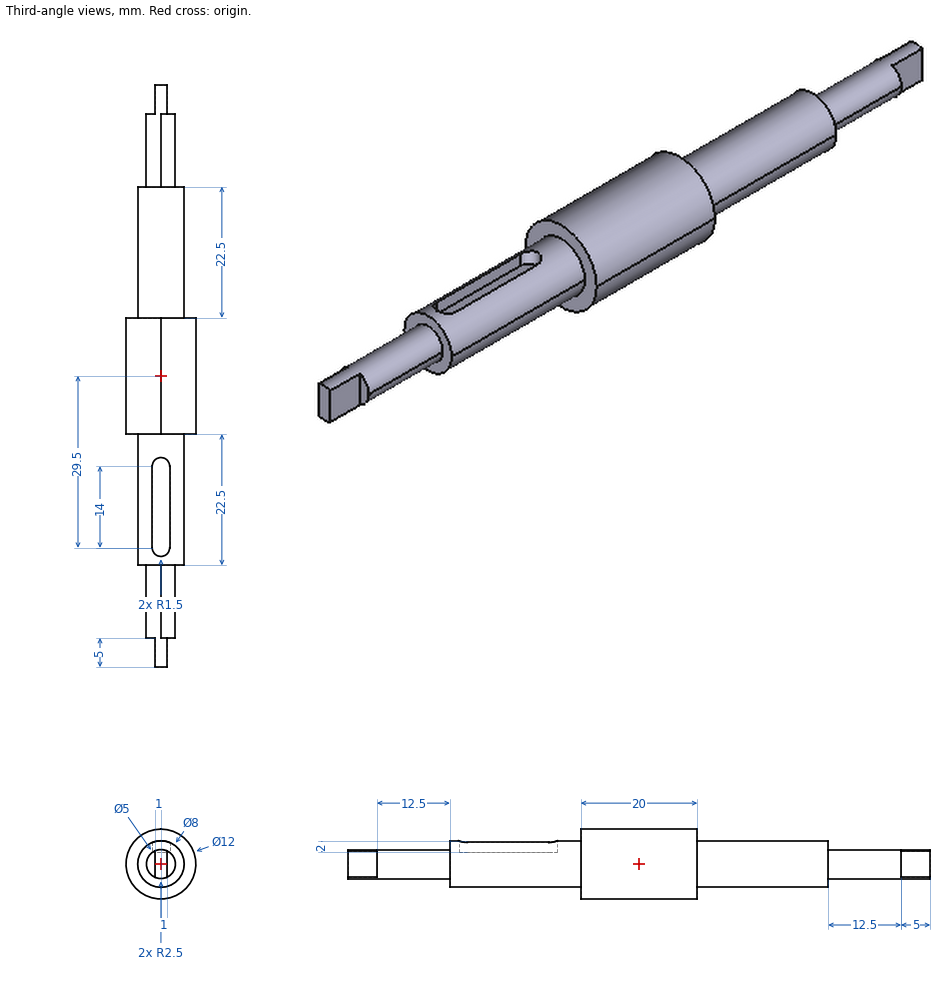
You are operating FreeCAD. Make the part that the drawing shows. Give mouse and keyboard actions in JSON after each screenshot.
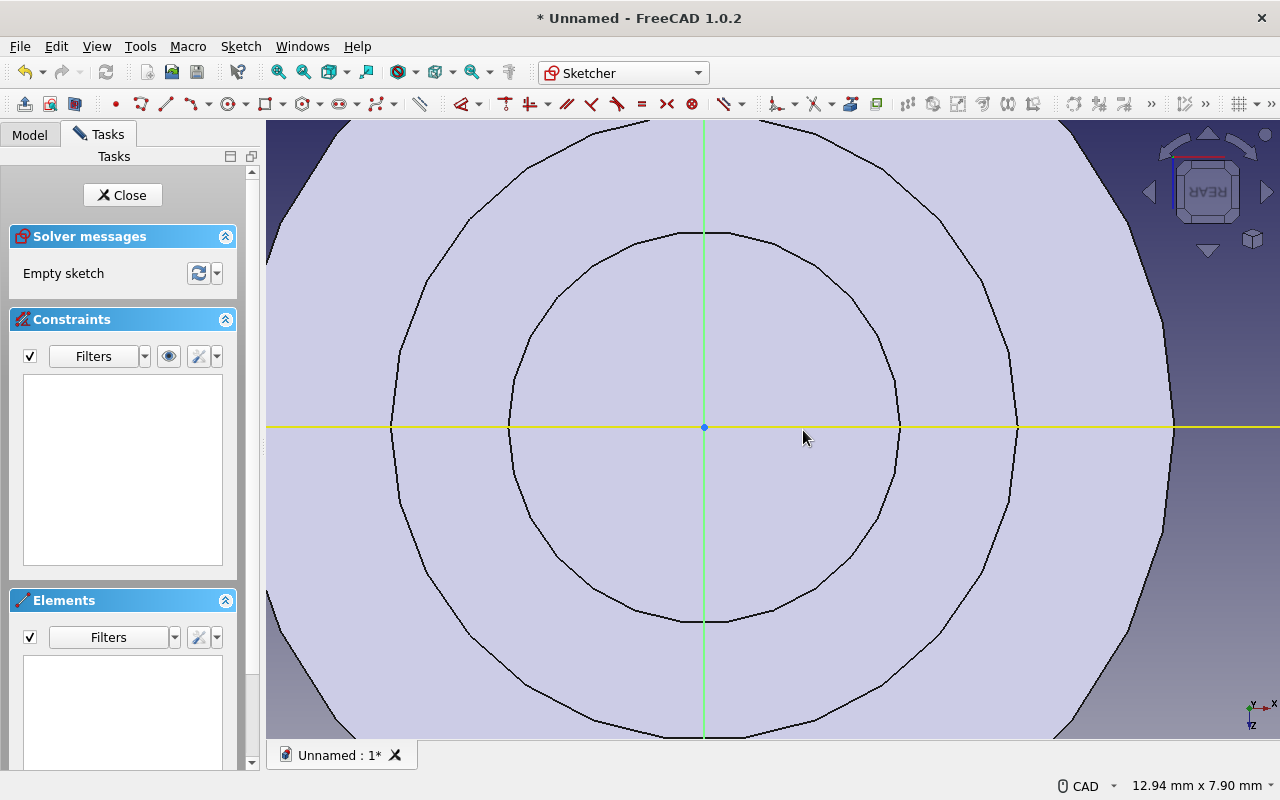
{"action": "key", "text": "g l"}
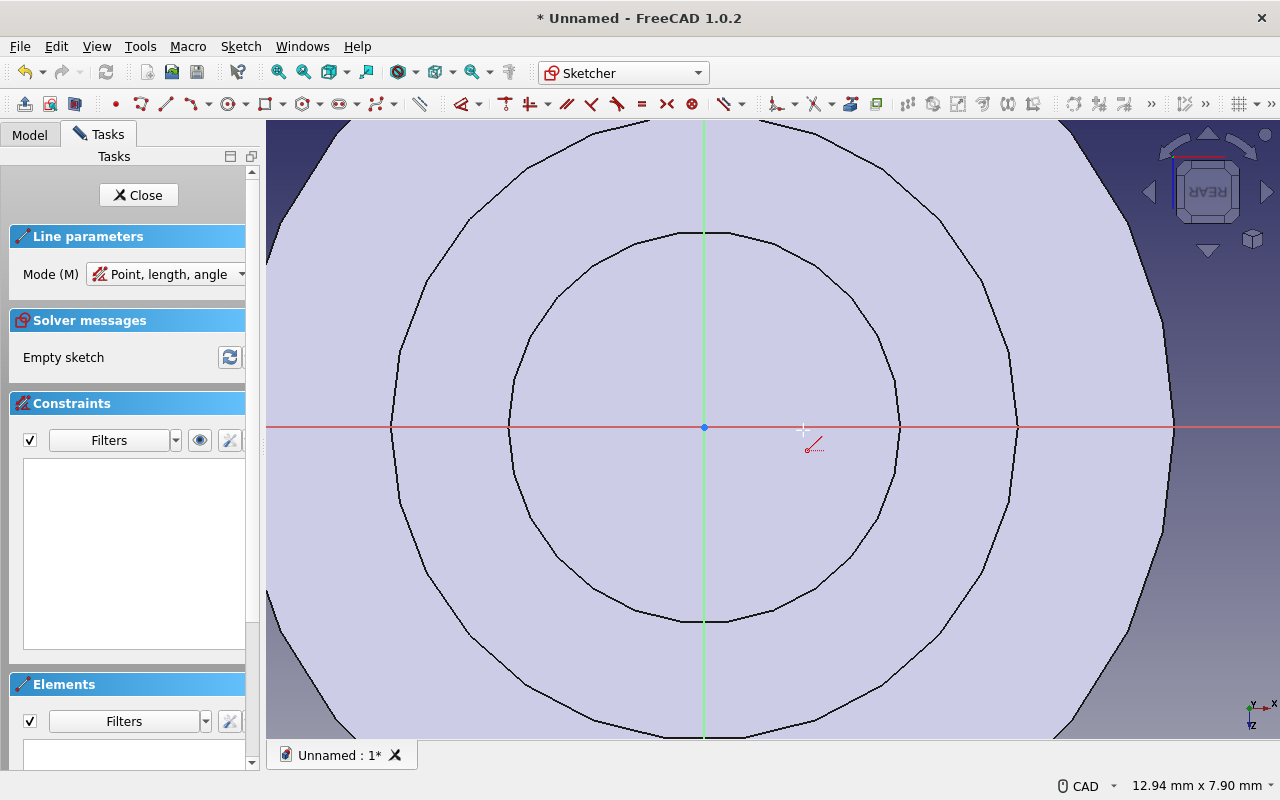
{"action": "left_click", "coordinate": [626, 248]}
{"action": "left_click", "coordinate": [626, 607]}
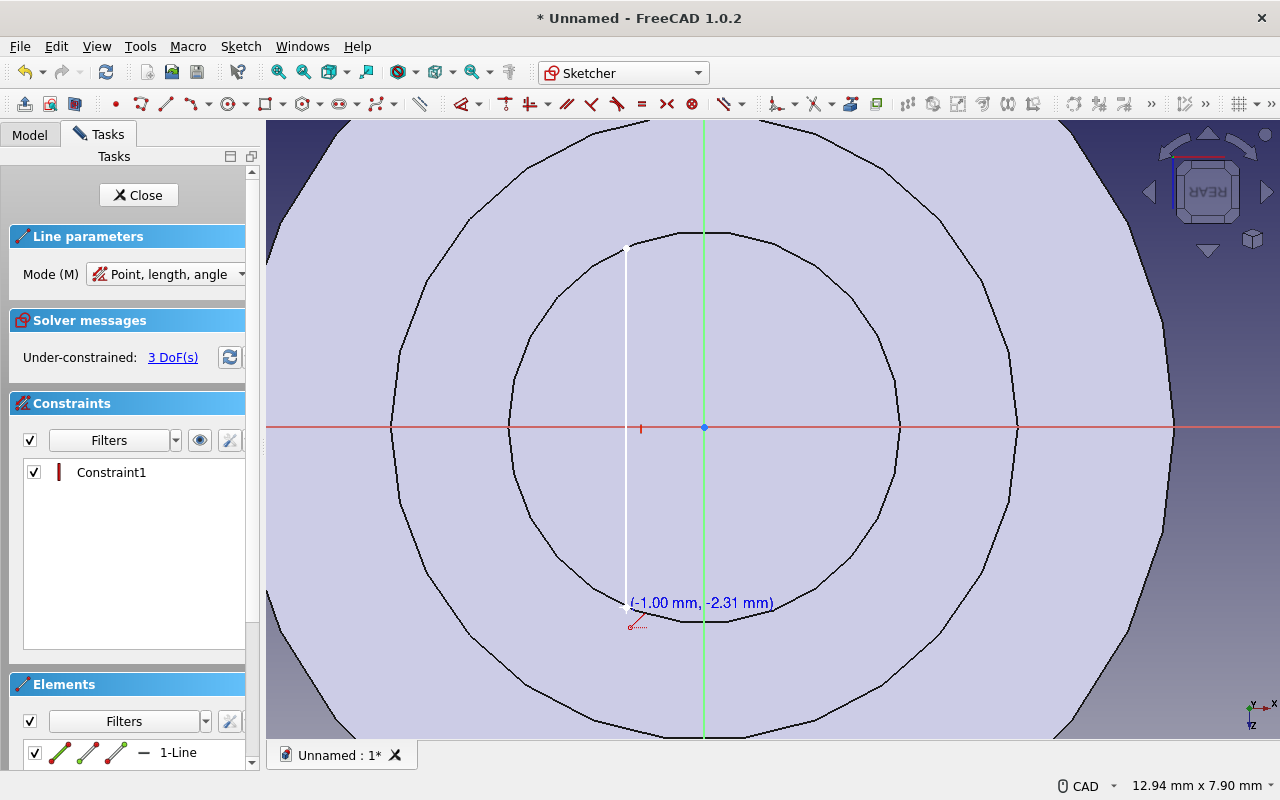
{"action": "left_click", "coordinate": [783, 607]}
{"action": "left_click", "coordinate": [783, 248]}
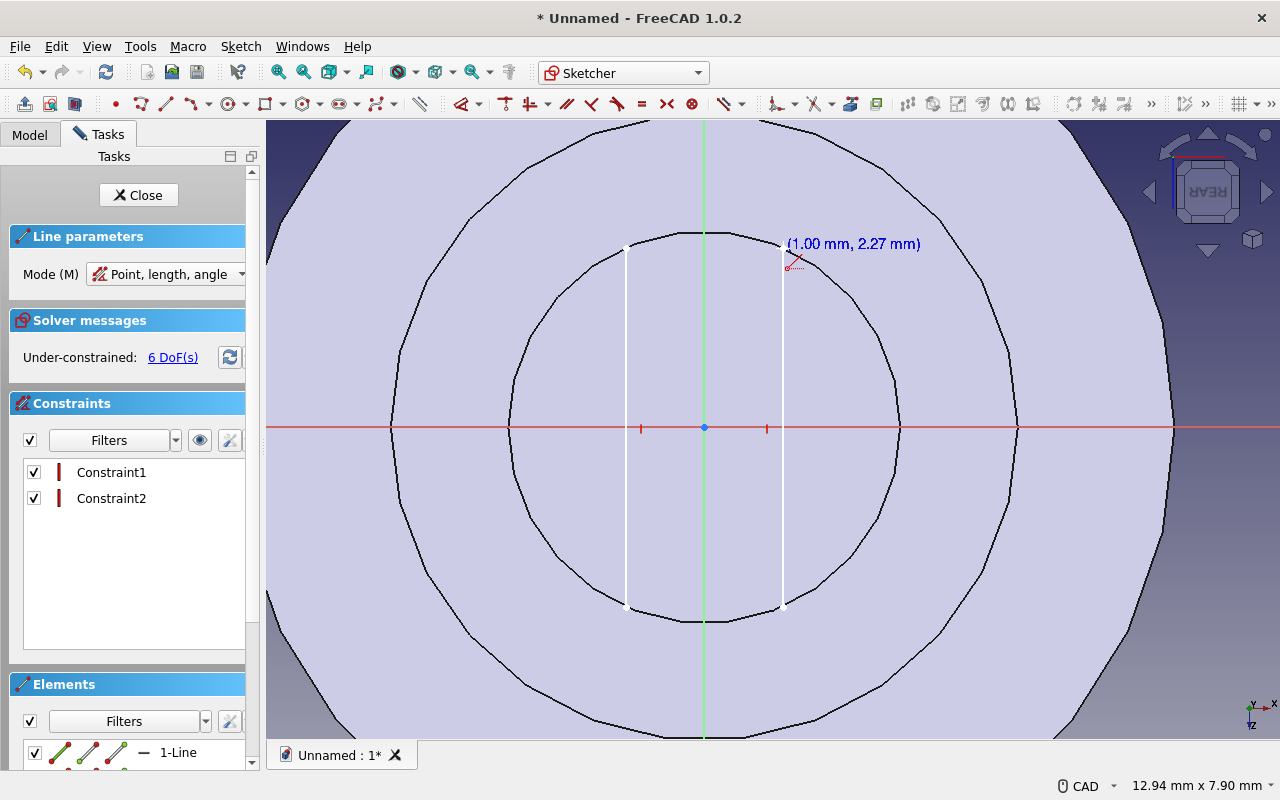
{"action": "key", "text": "g 3 a"}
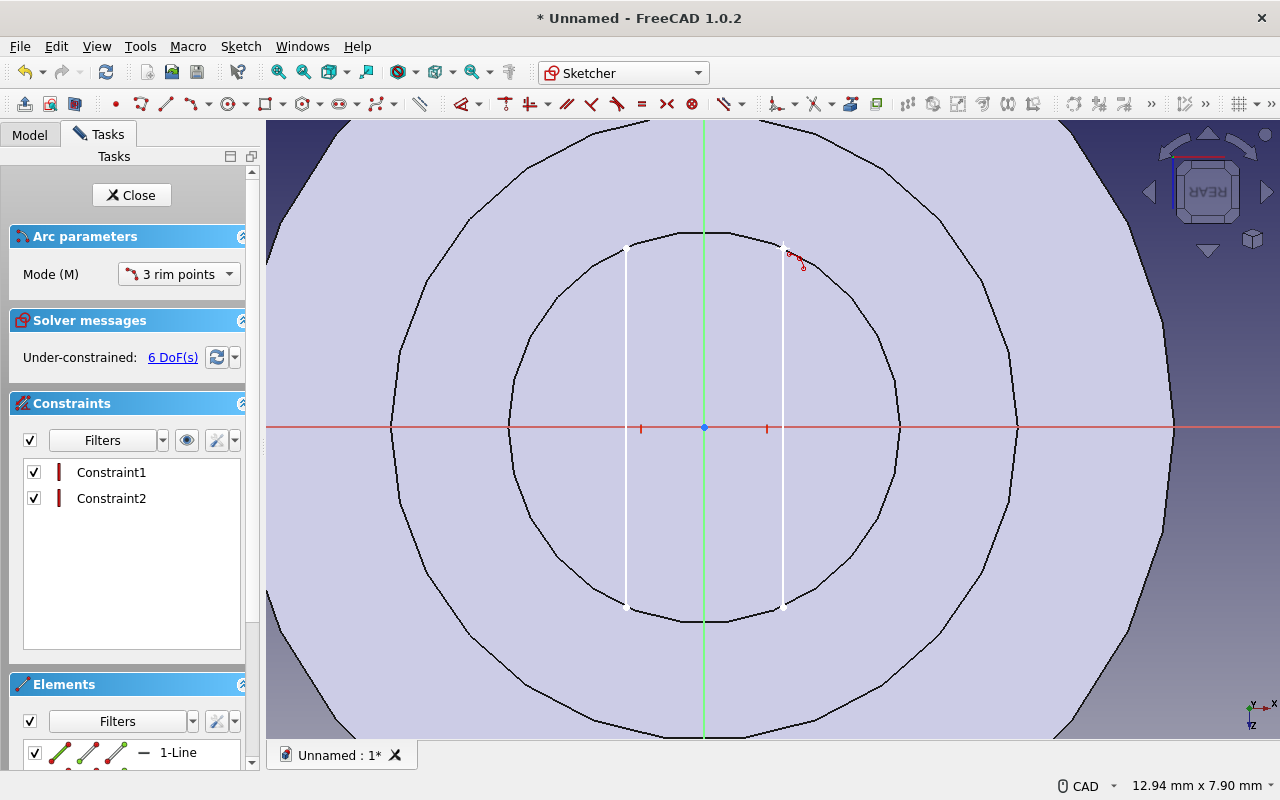
{"action": "left_click", "coordinate": [626, 608]}
{"action": "left_click", "coordinate": [783, 608]}
{"action": "left_click", "coordinate": [688, 622]}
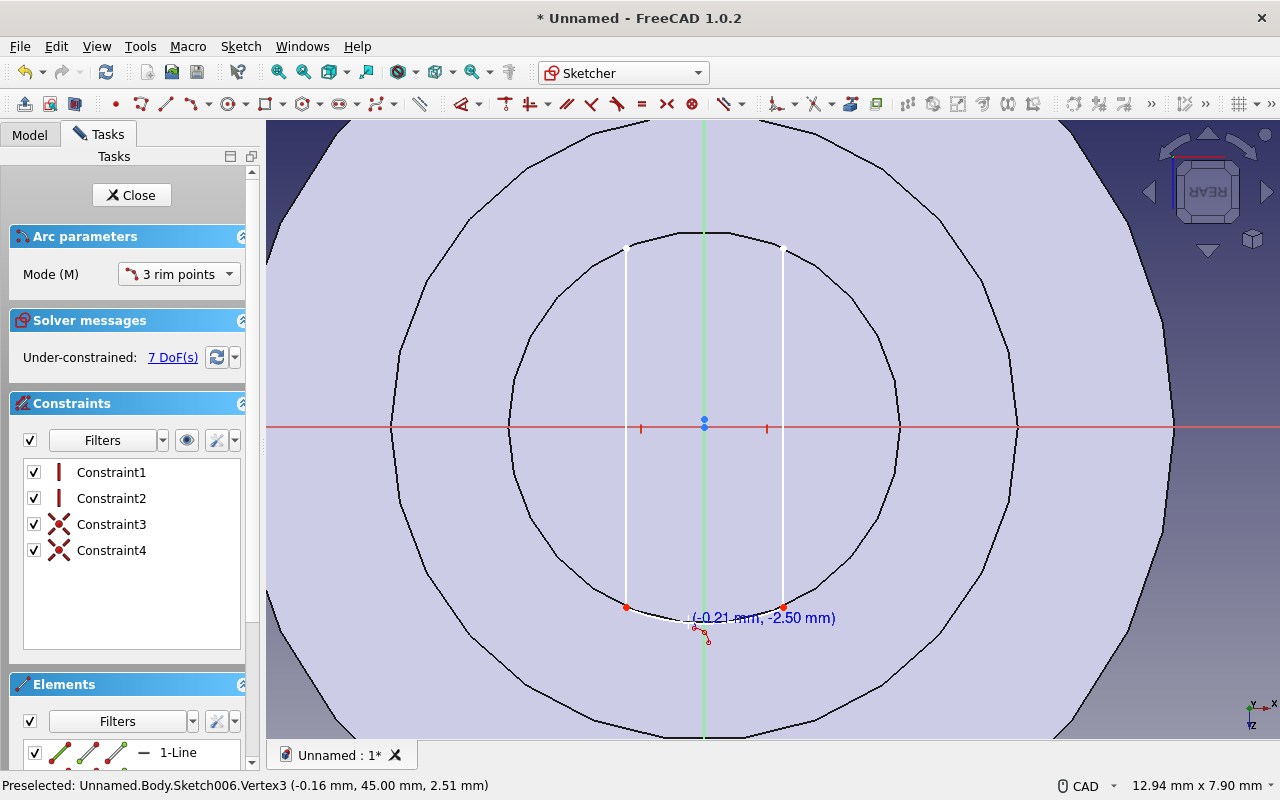
{"action": "left_click", "coordinate": [783, 249]}
{"action": "left_click", "coordinate": [626, 249]}
{"action": "left_click", "coordinate": [720, 232]}
{"action": "key", "text": "Escape"}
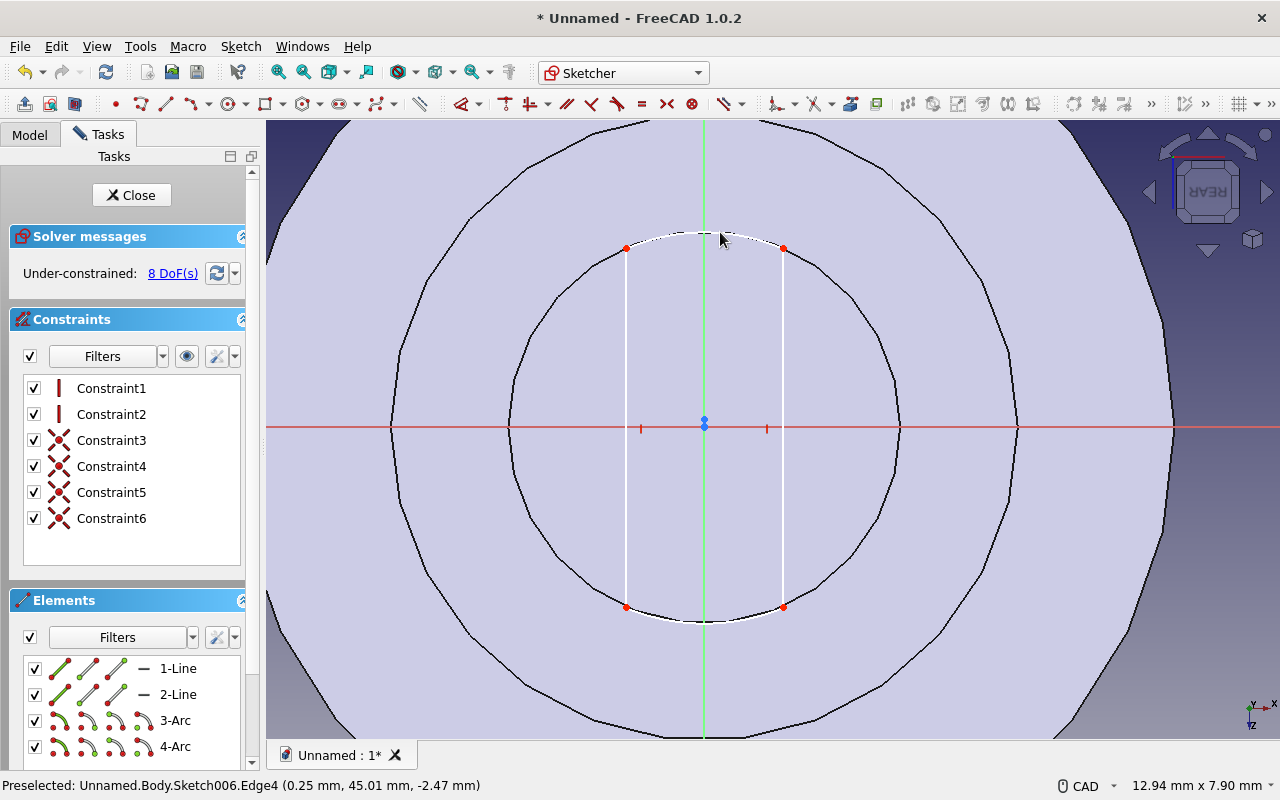
{"action": "left_click", "coordinate": [672, 621]}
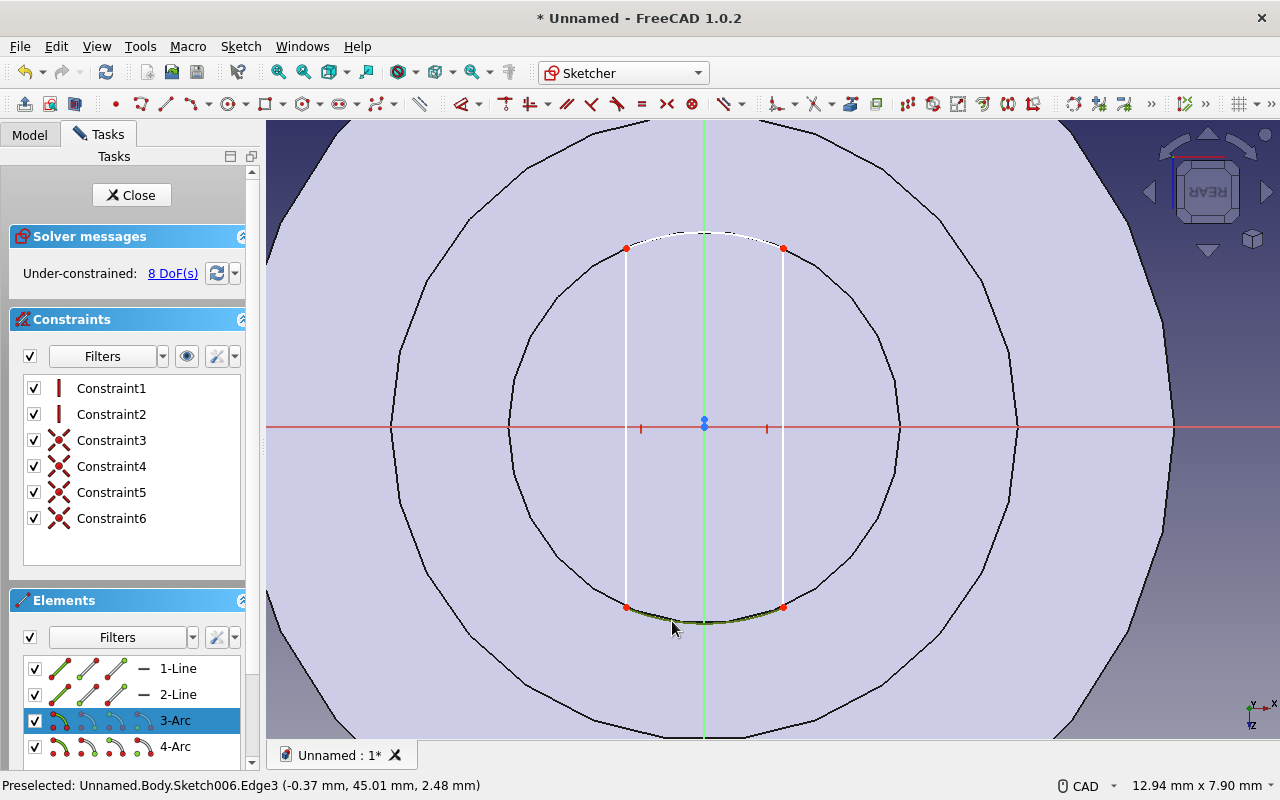
{"action": "left_click", "coordinate": [737, 235]}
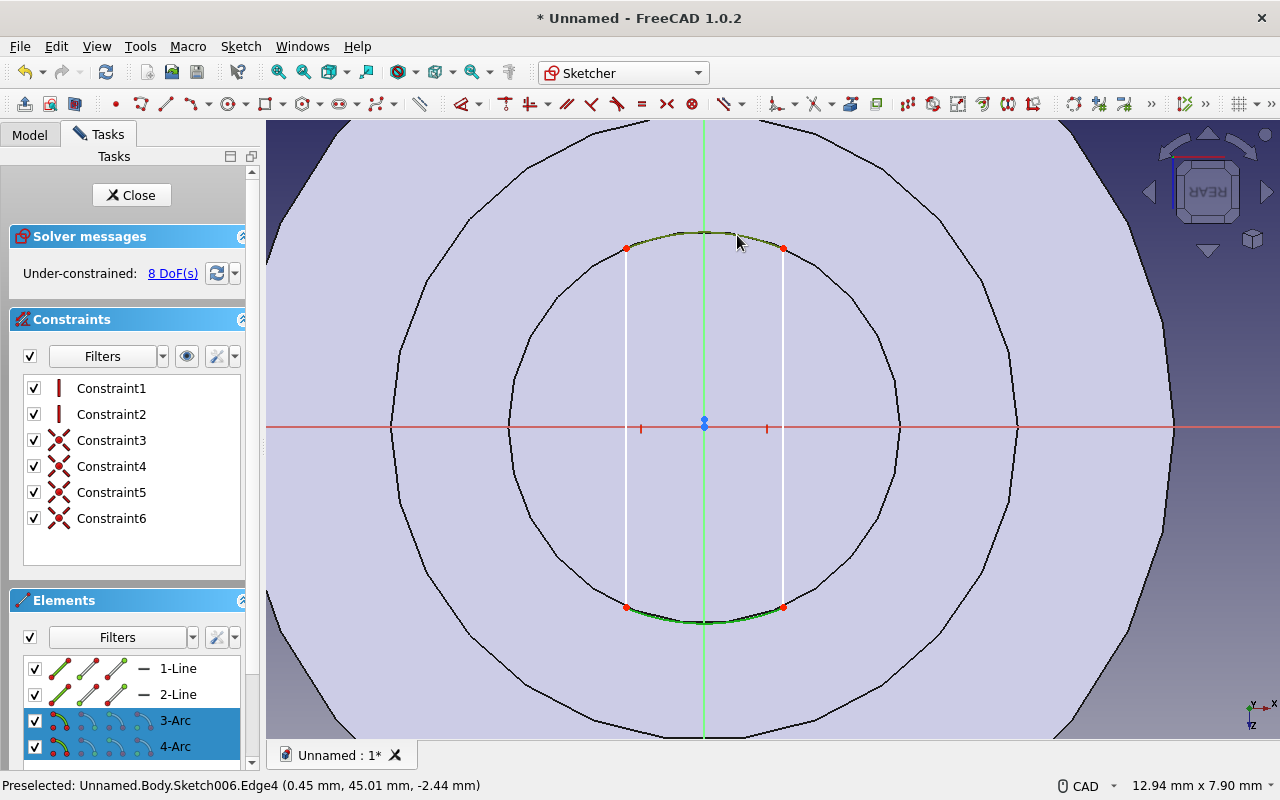
{"action": "left_click", "coordinate": [505, 104]}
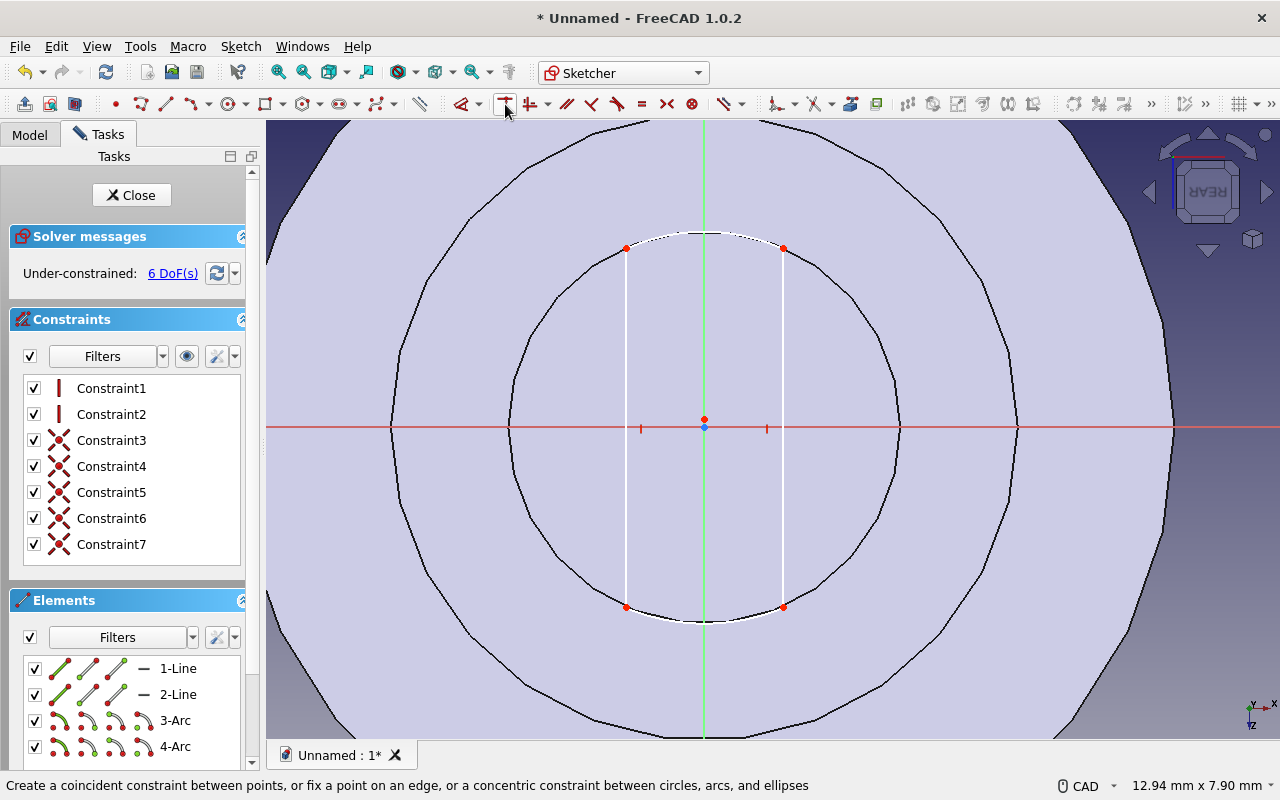
{"action": "left_click_drag", "start_coordinate": [694, 409], "coordinate": [714, 437]}